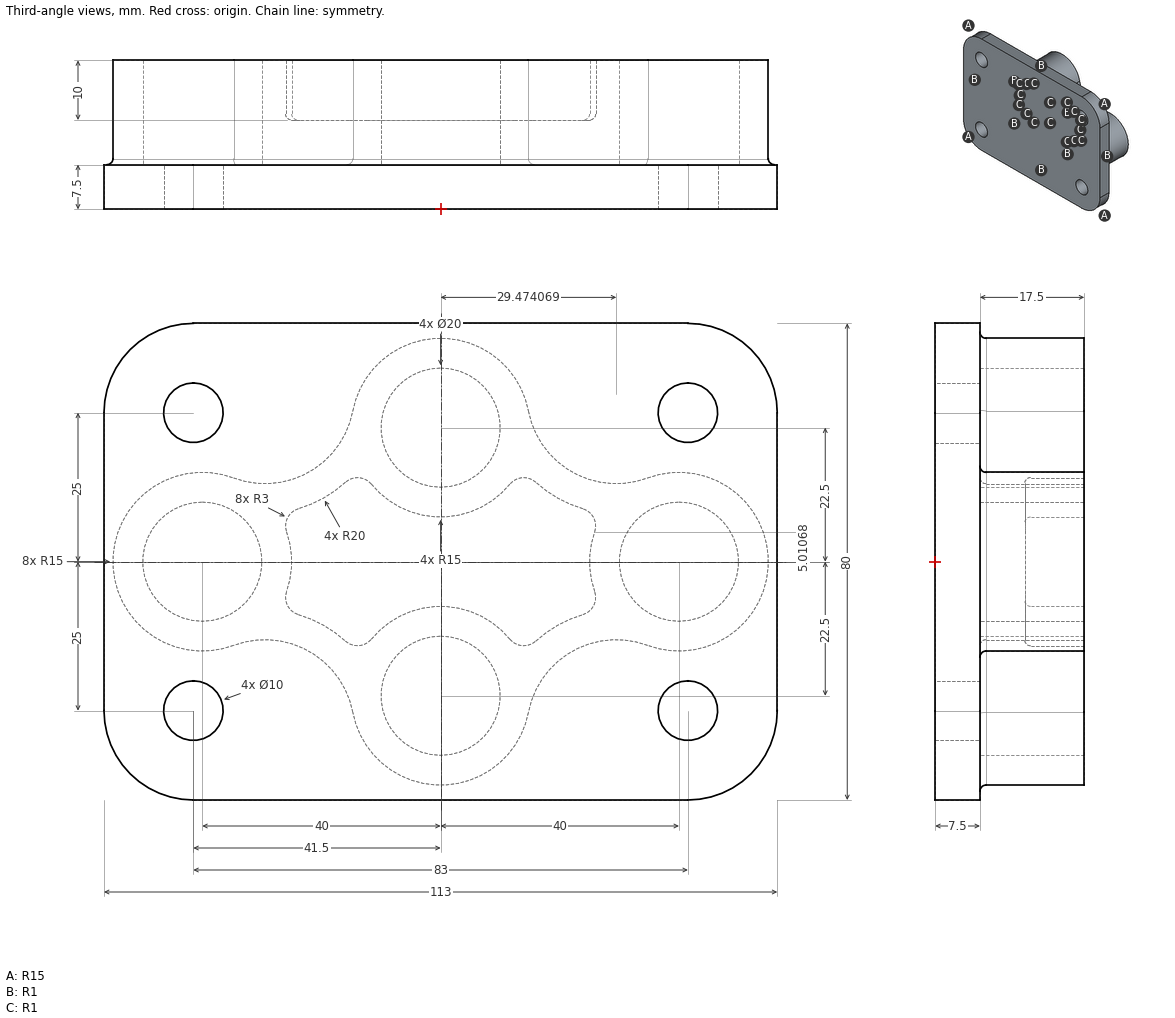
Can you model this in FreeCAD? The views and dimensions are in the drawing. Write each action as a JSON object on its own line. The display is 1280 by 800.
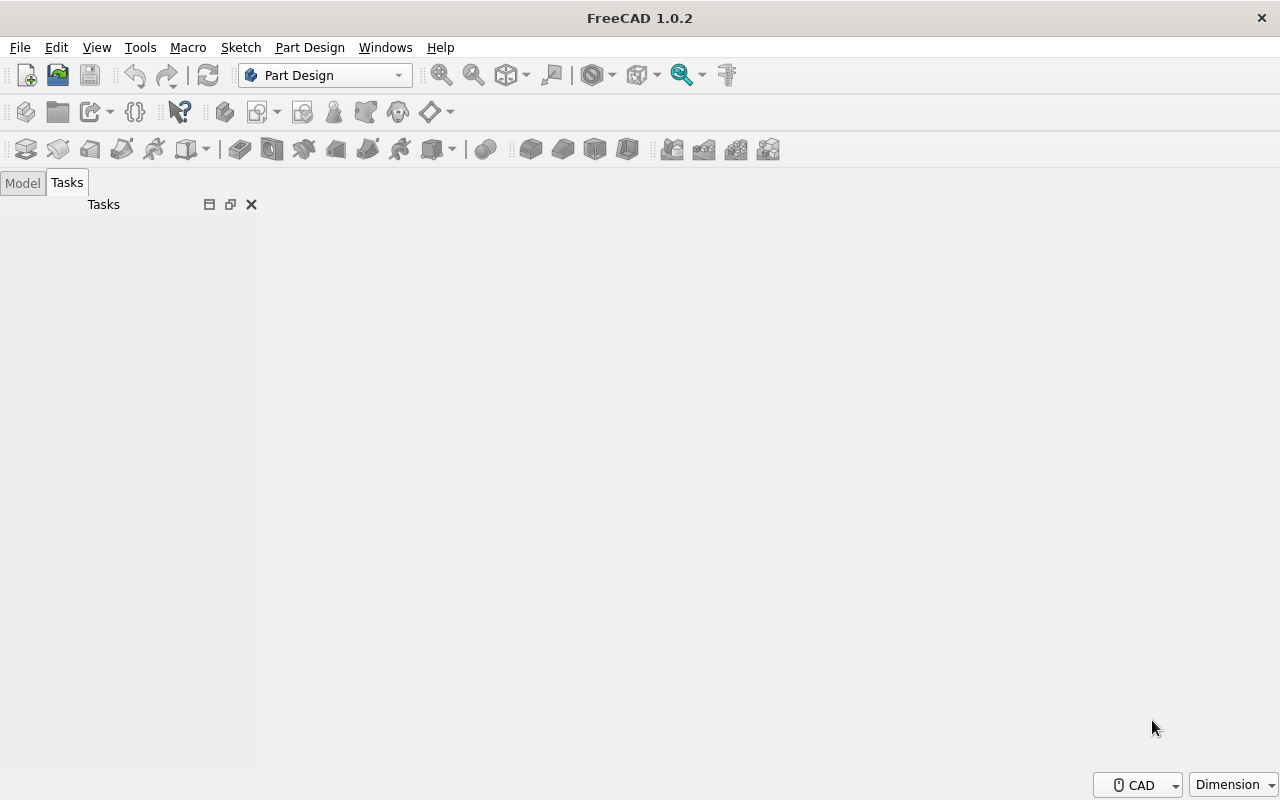
{"action": "key", "text": "ctrl+n"}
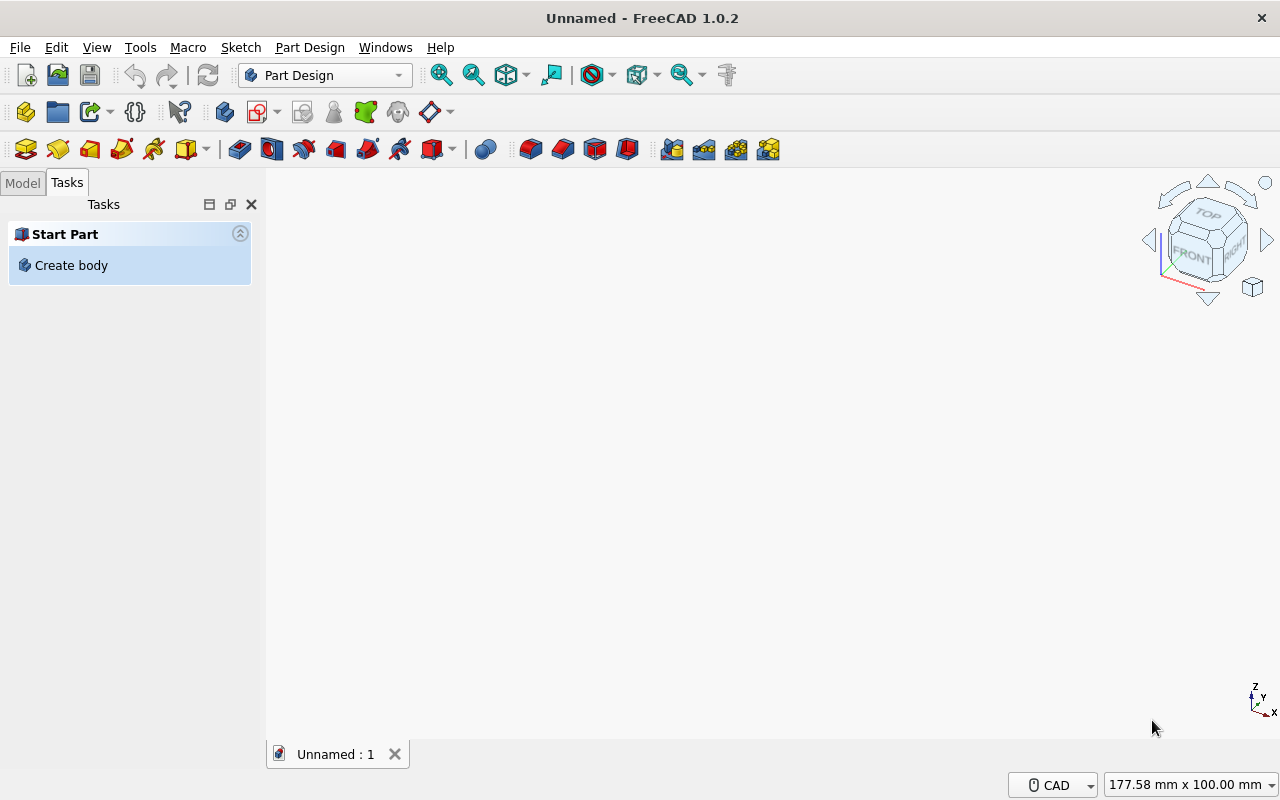
{"action": "left_click", "coordinate": [258, 112]}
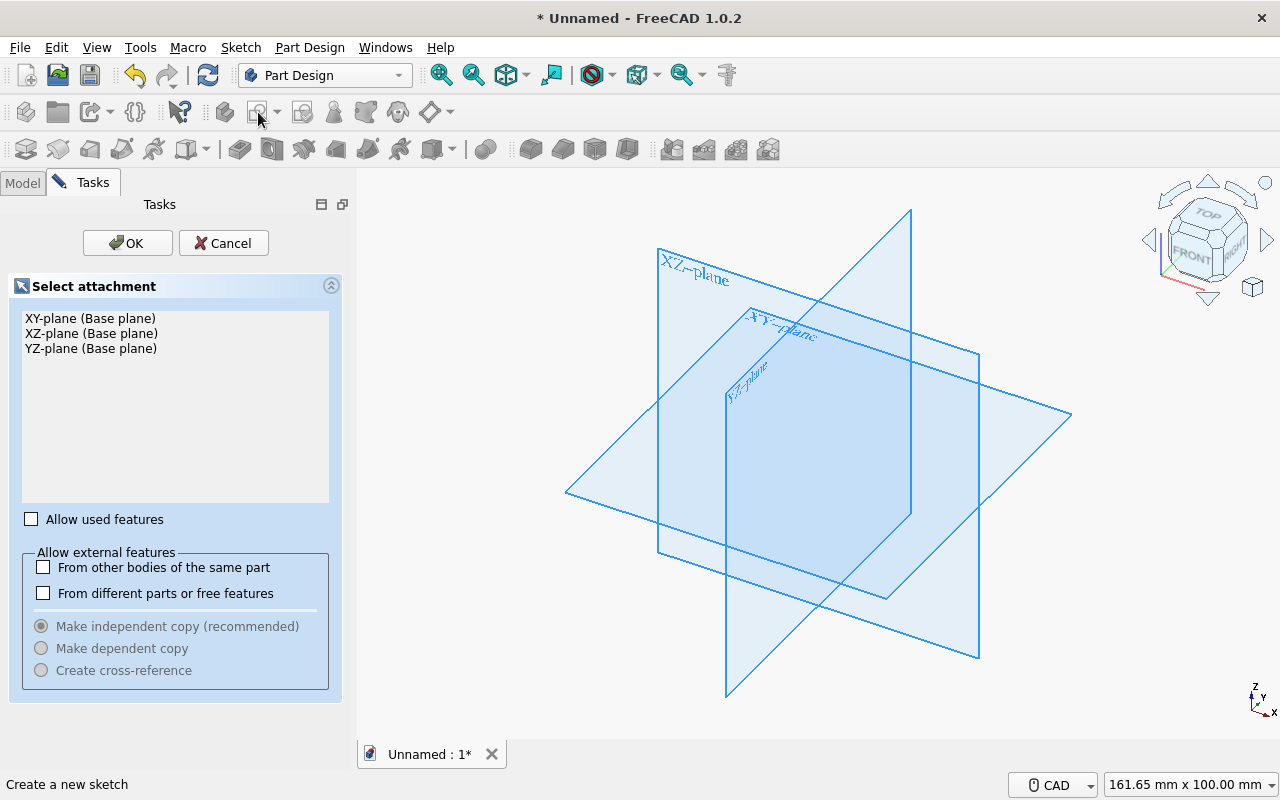
{"action": "left_click", "coordinate": [82, 334]}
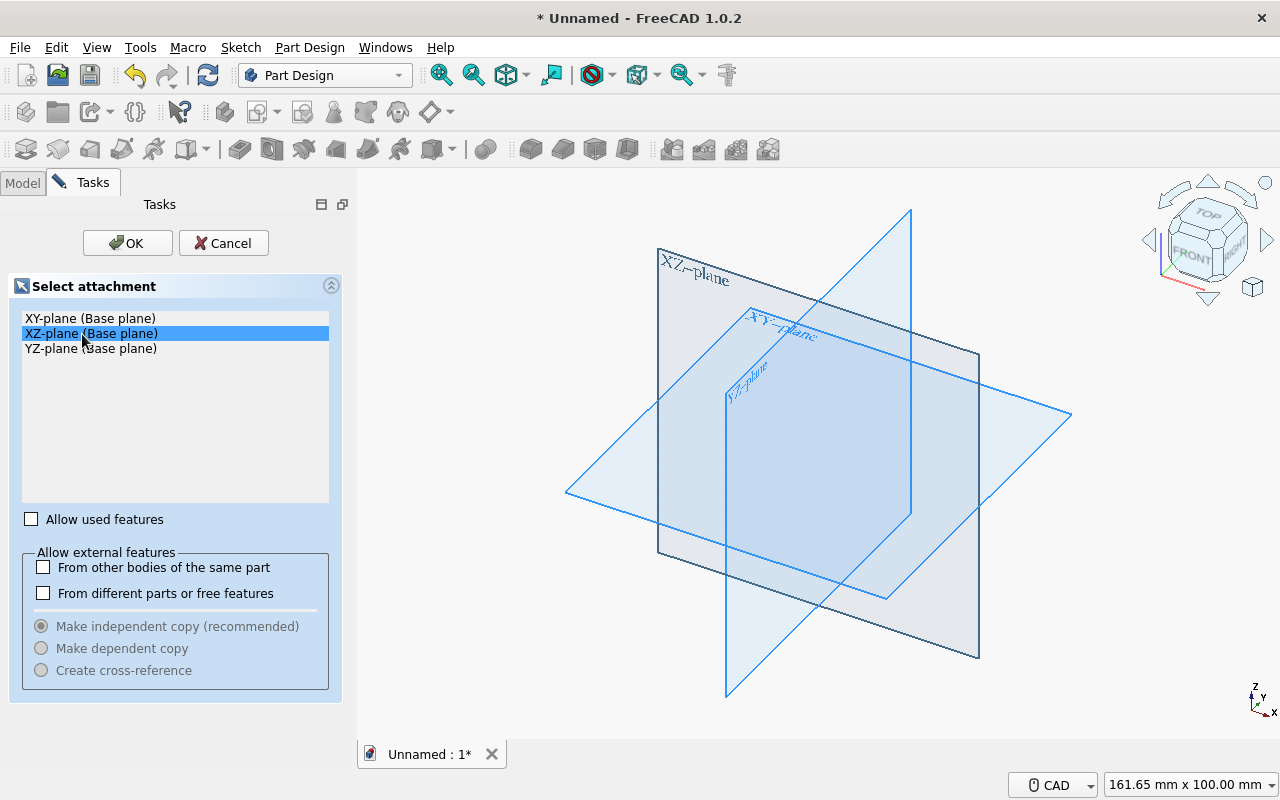
{"action": "left_click", "coordinate": [128, 243]}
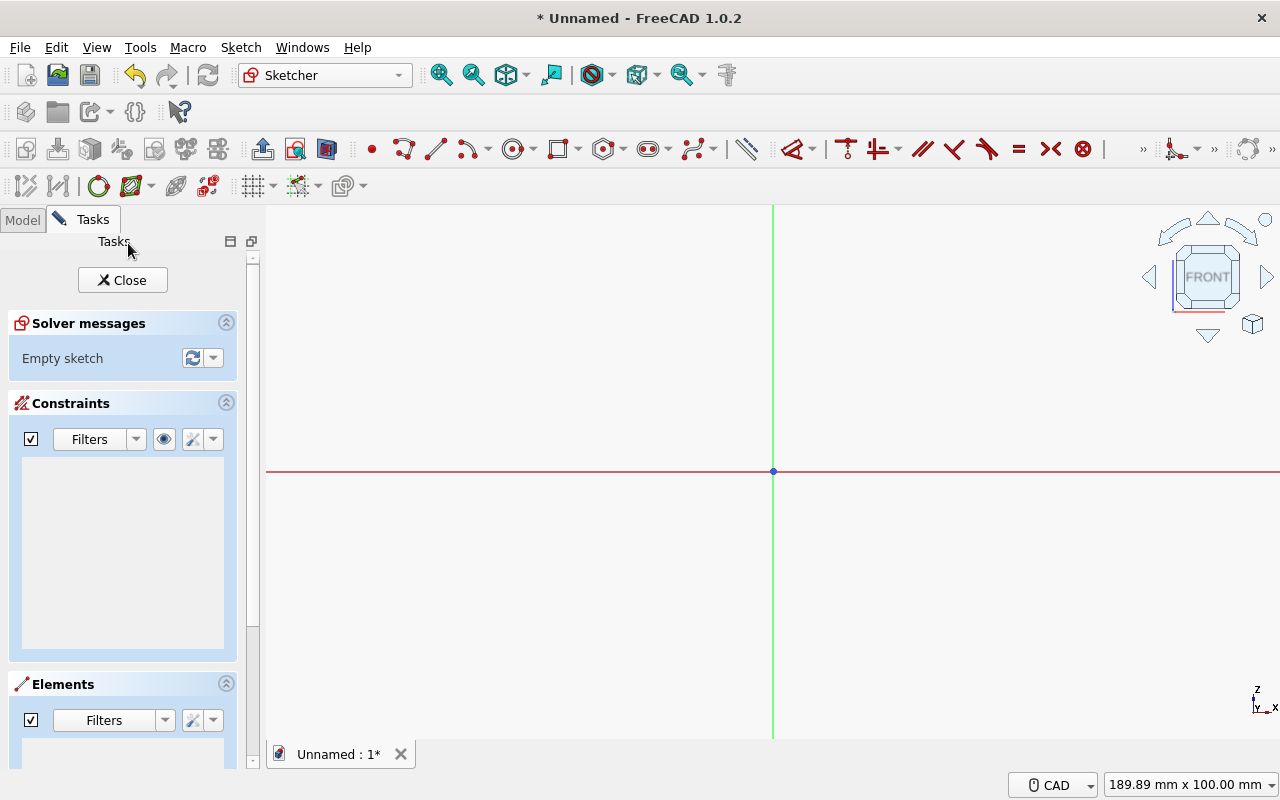
{"action": "key", "text": "g v"}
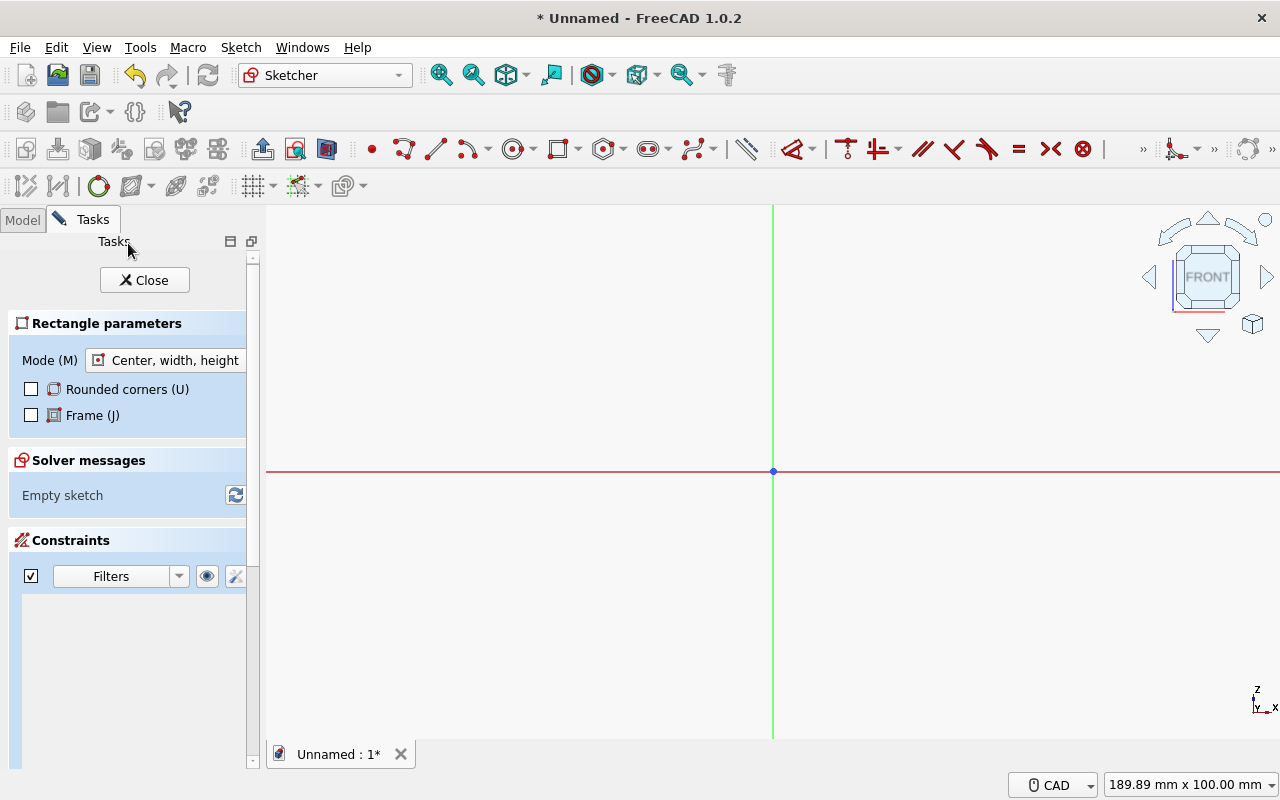
{"action": "left_click", "coordinate": [773, 472]}
{"action": "mouse_move", "coordinate": [1075, 258]}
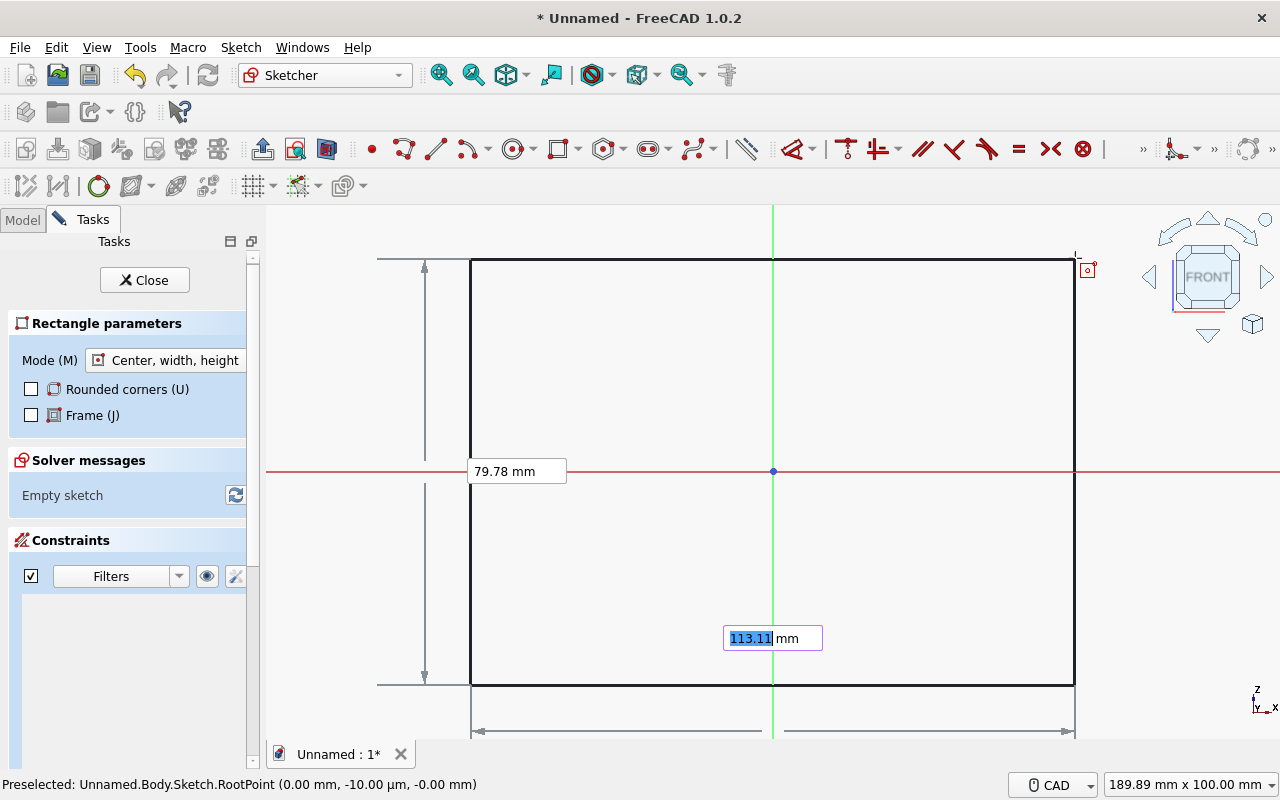
{"action": "type", "text": "113"}
{"action": "key", "text": "Tab"}
{"action": "type", "text": "80"}
{"action": "key", "text": "Return"}
{"action": "key", "text": "Escape"}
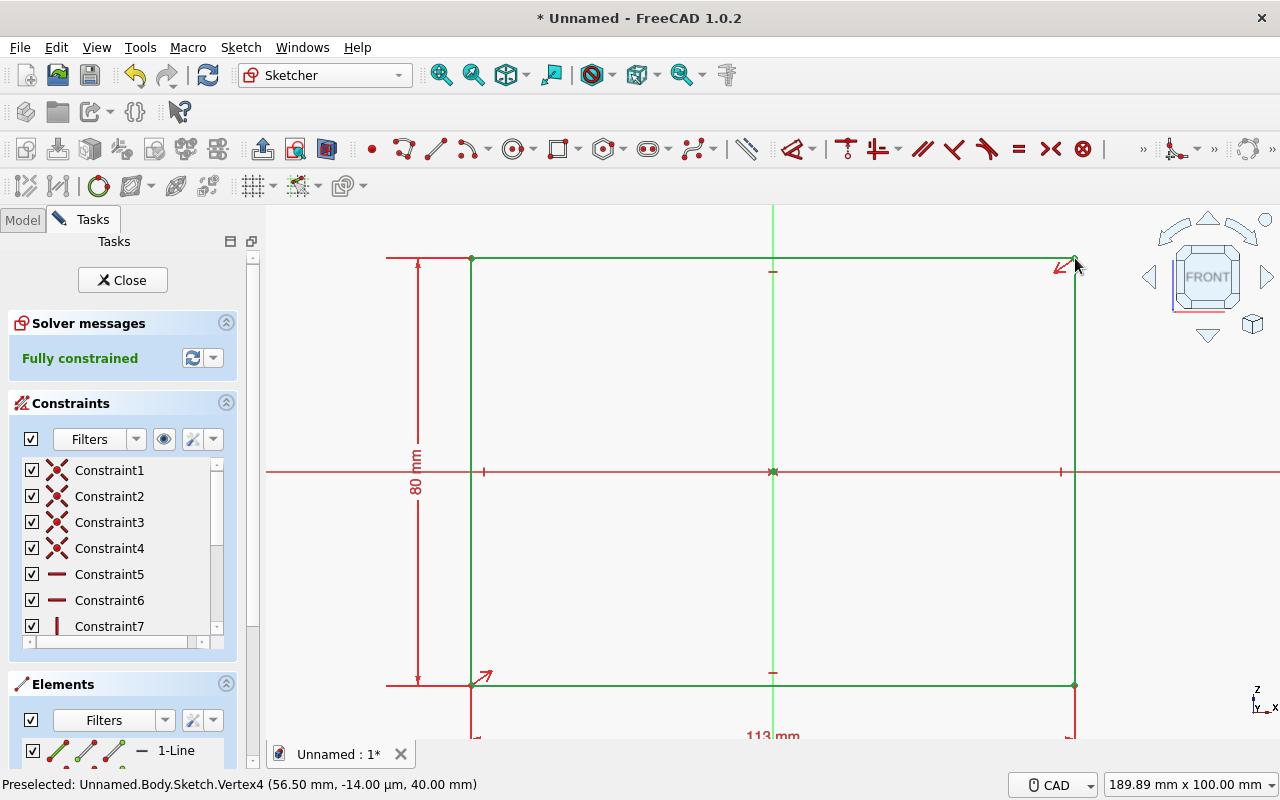
{"action": "left_click", "coordinate": [123, 280]}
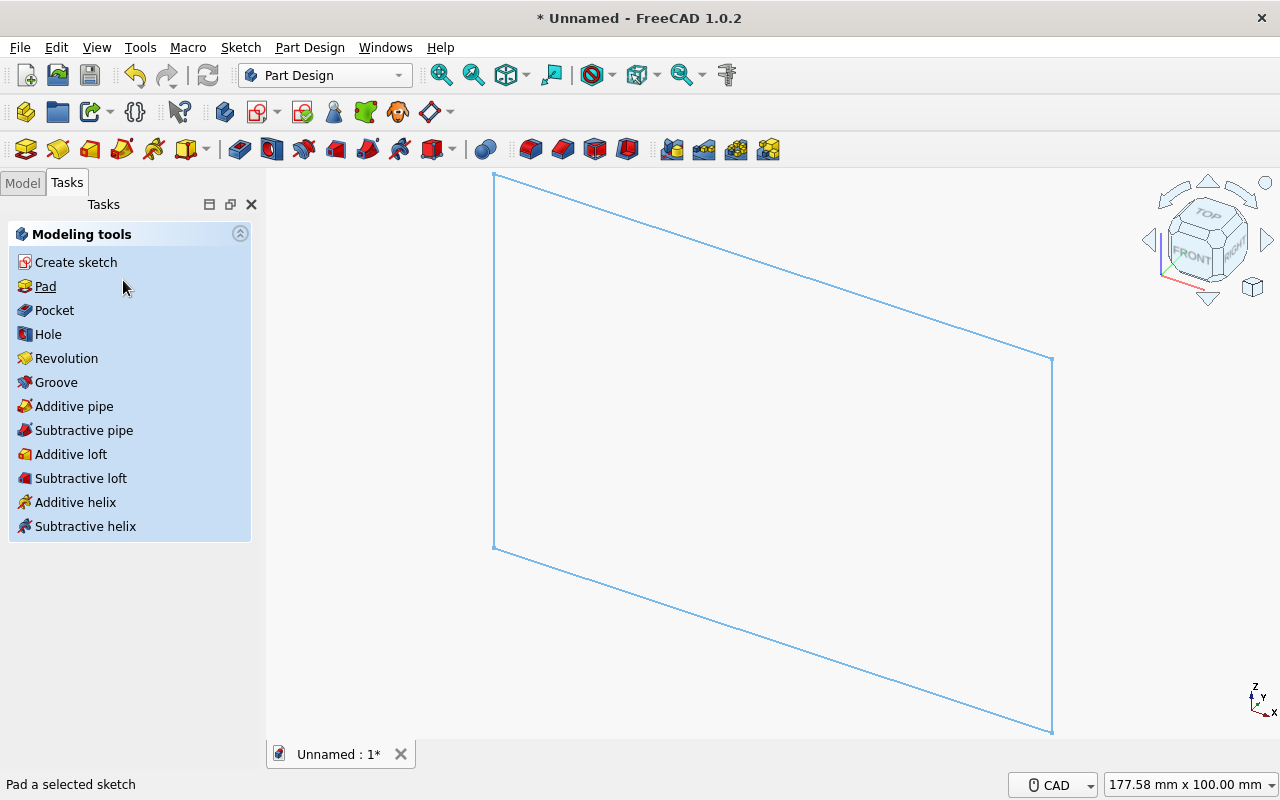
{"action": "left_click", "coordinate": [26, 150]}